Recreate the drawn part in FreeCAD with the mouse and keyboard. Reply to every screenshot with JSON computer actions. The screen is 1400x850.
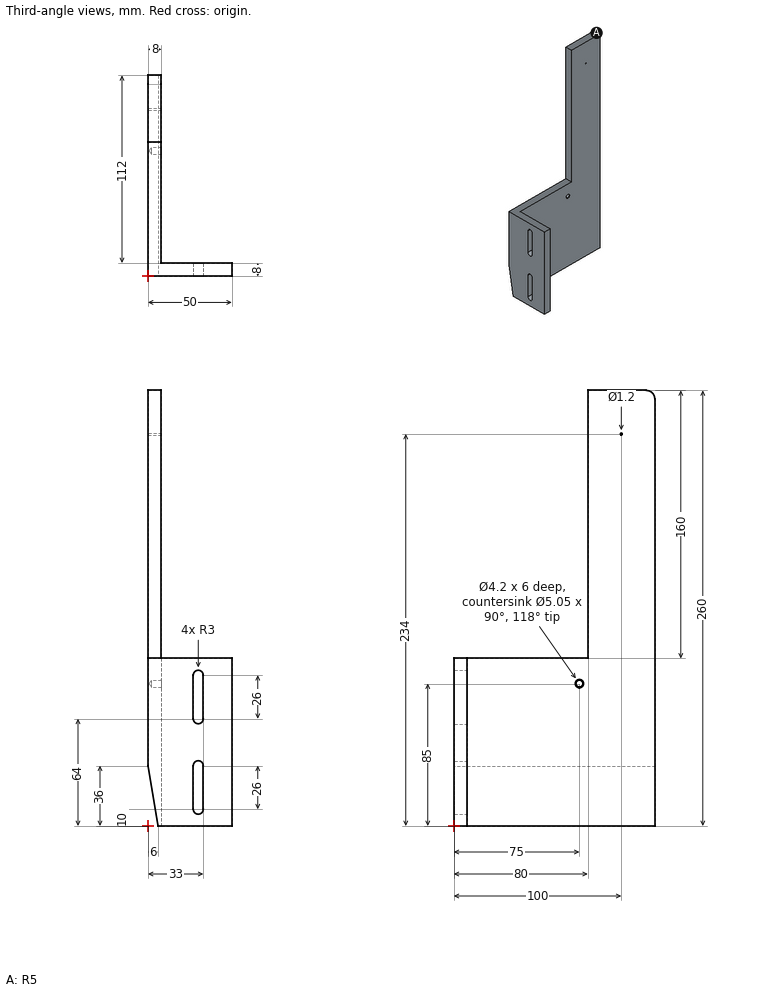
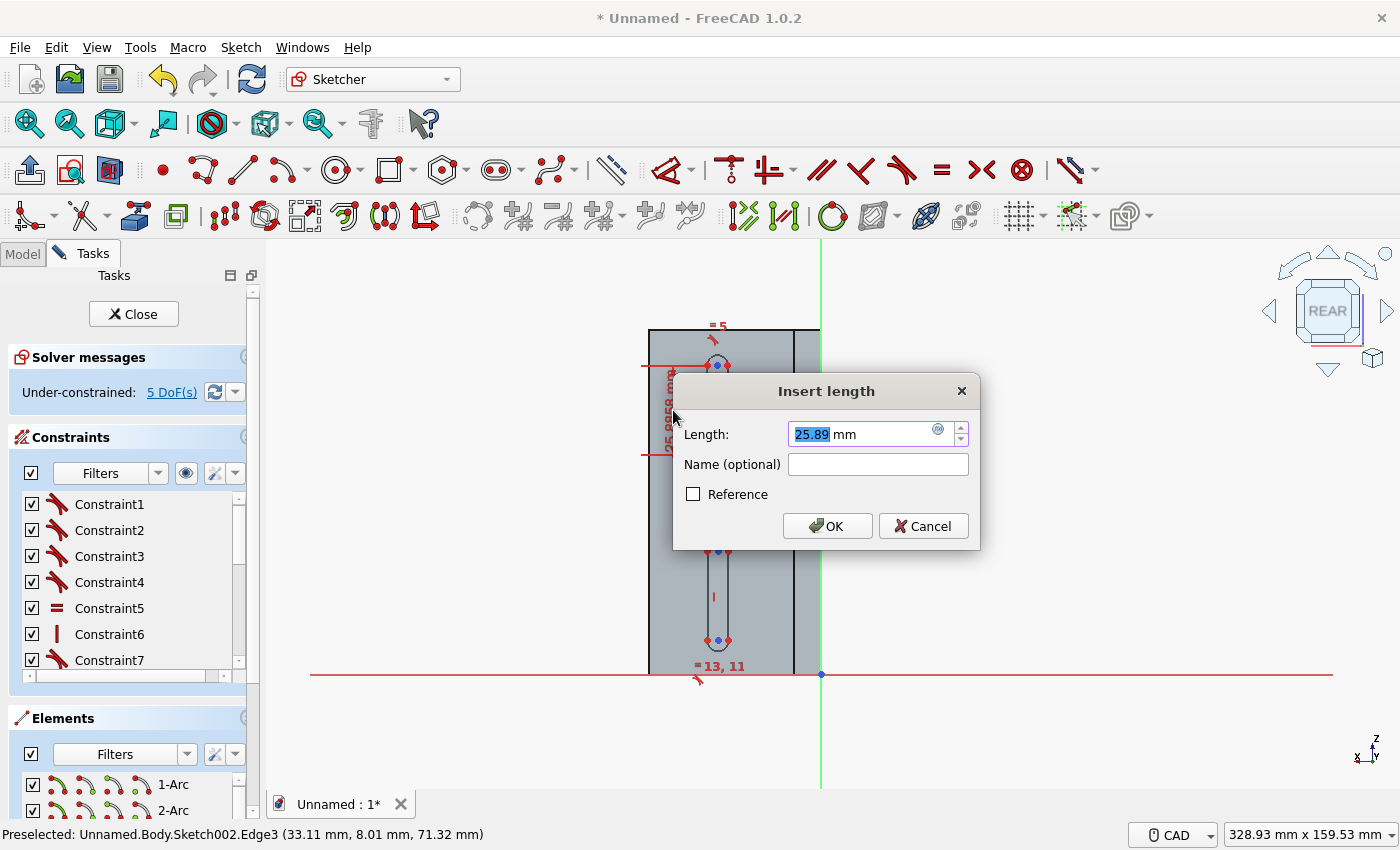
{"action": "type", "text": "26"}
{"action": "key", "text": "Return"}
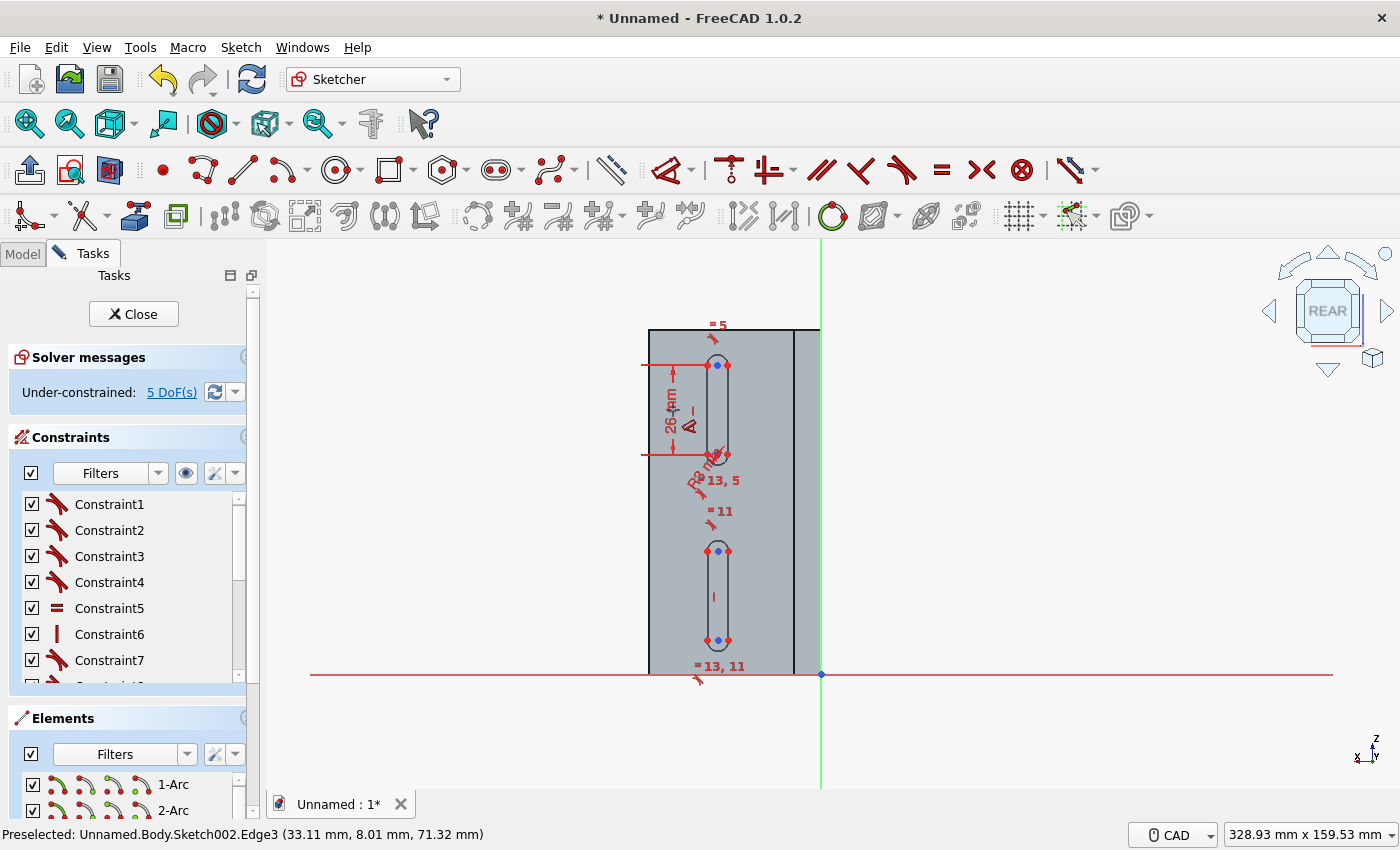
{"action": "left_click", "coordinate": [708, 614]}
{"action": "left_click", "coordinate": [674, 596]}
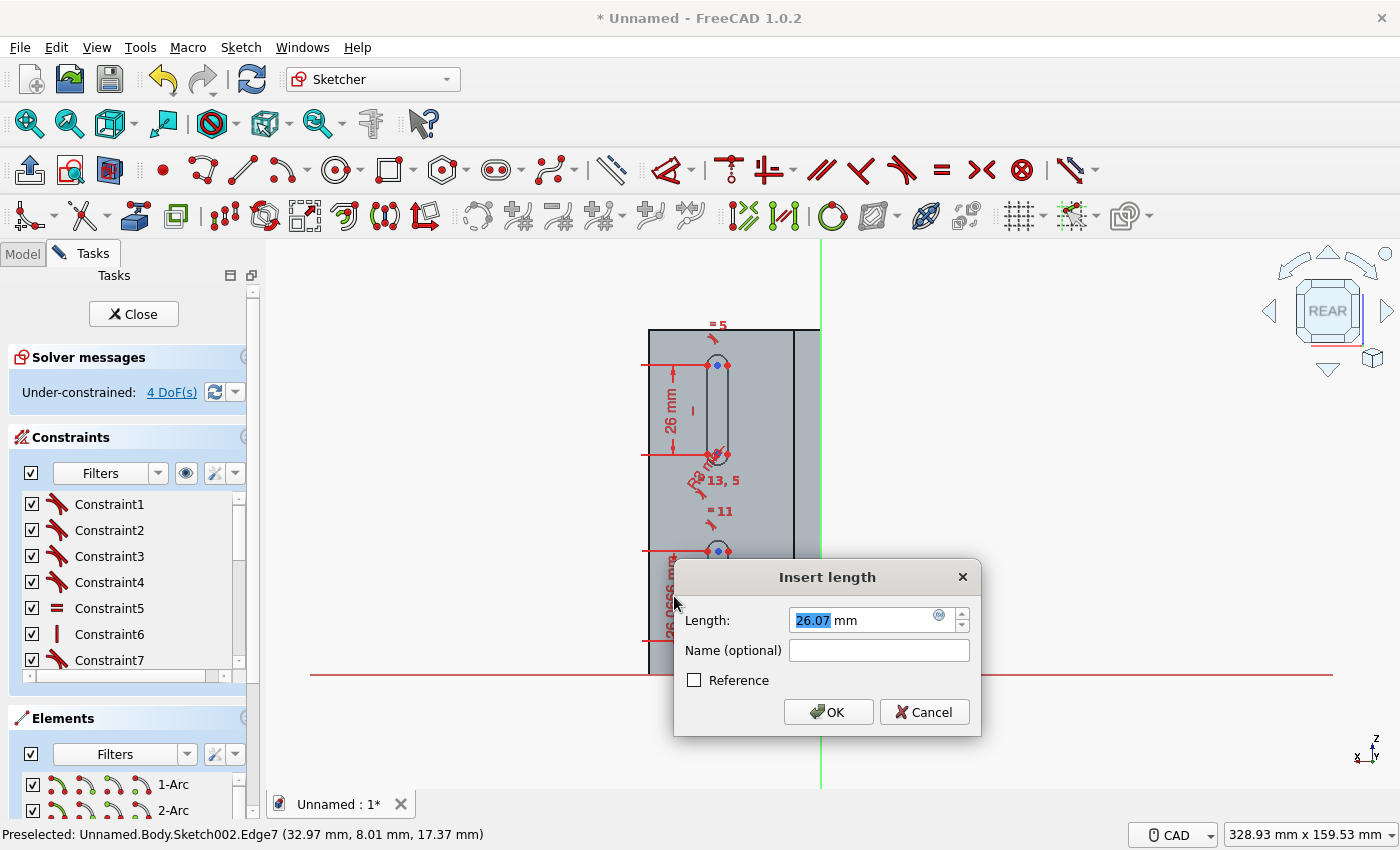
{"action": "type", "text": "26"}
{"action": "key", "text": "Return"}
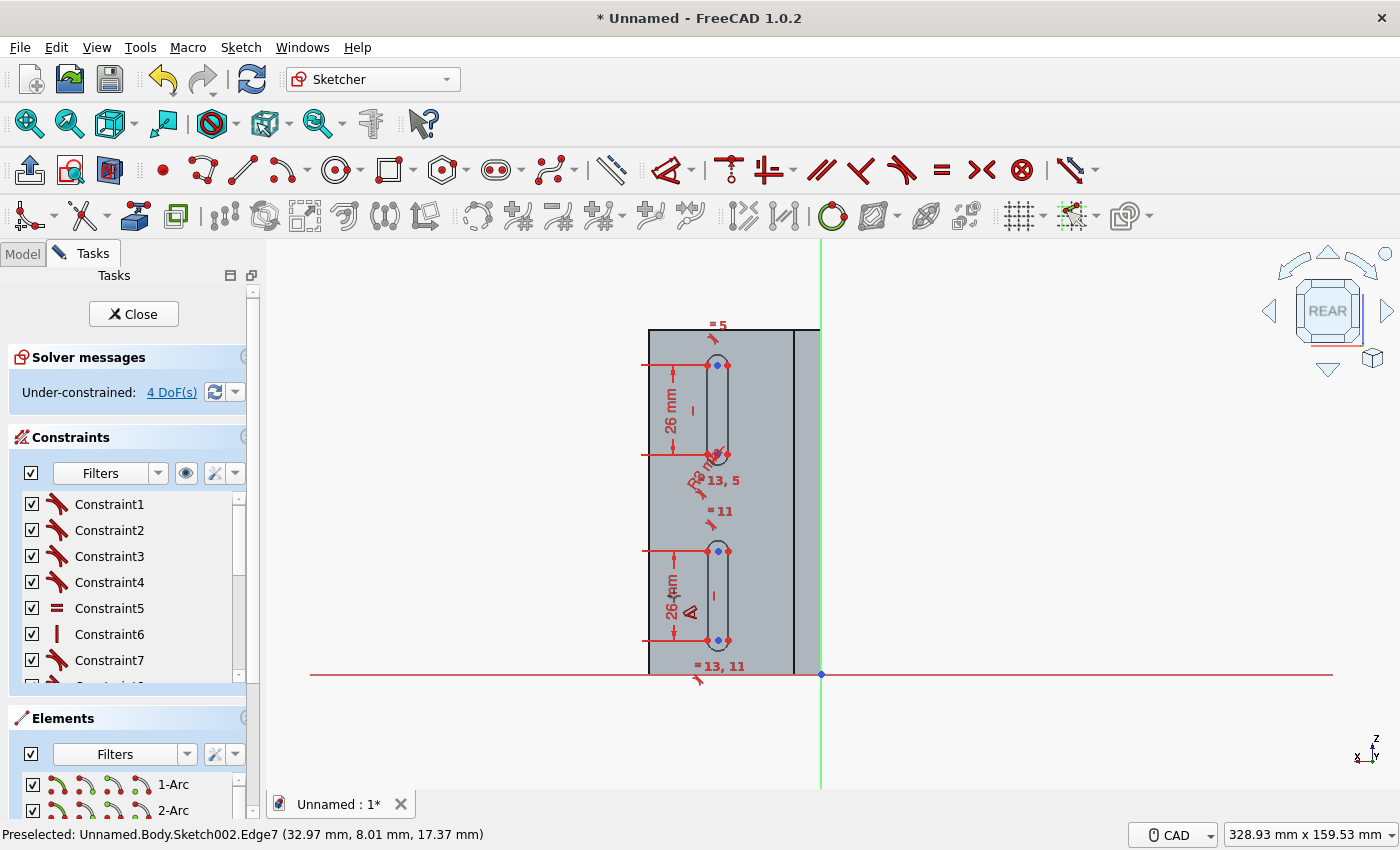
{"action": "left_click", "coordinate": [707, 455]}
{"action": "left_click", "coordinate": [764, 709]}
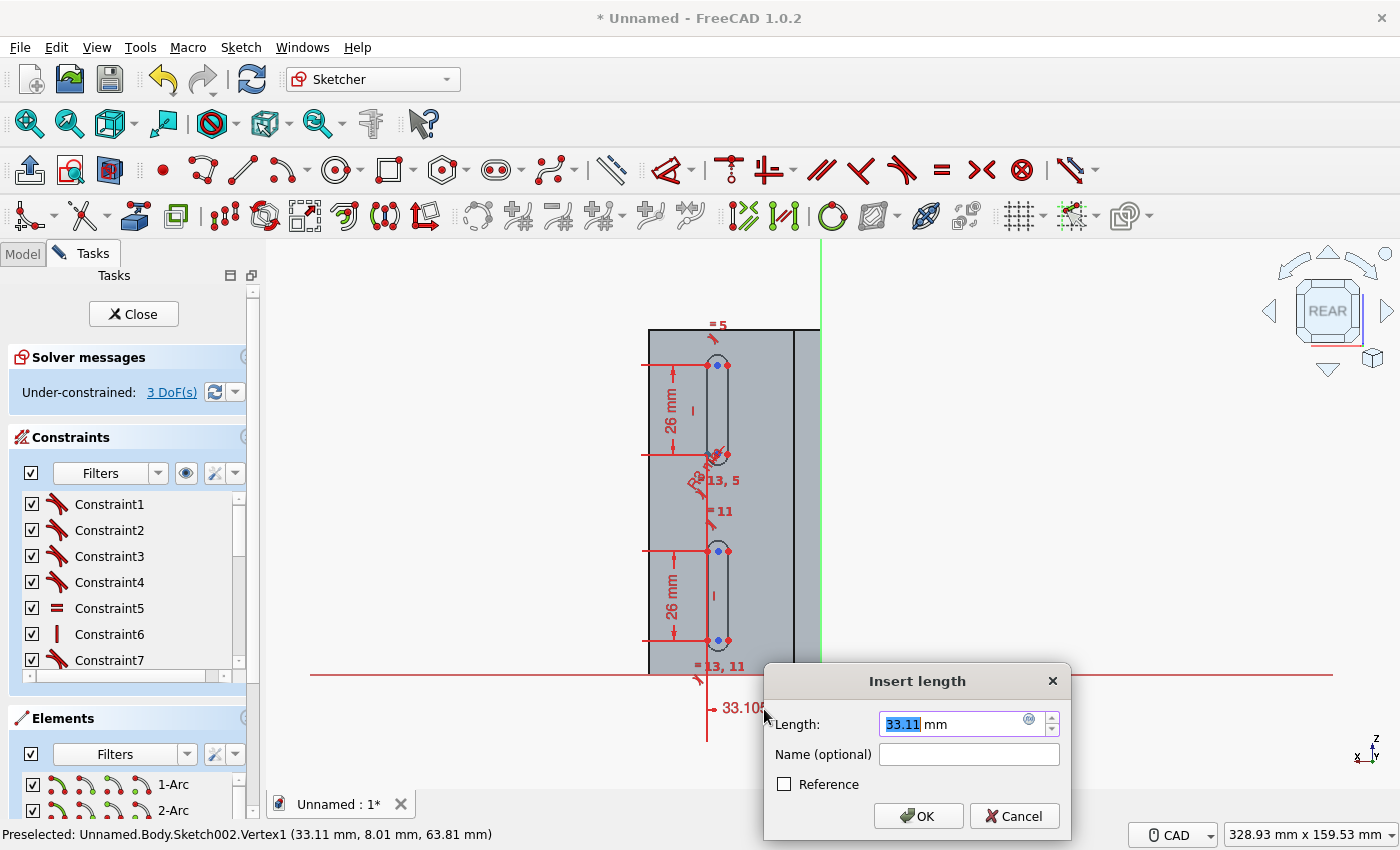
{"action": "type", "text": "33"}
{"action": "key", "text": "Return"}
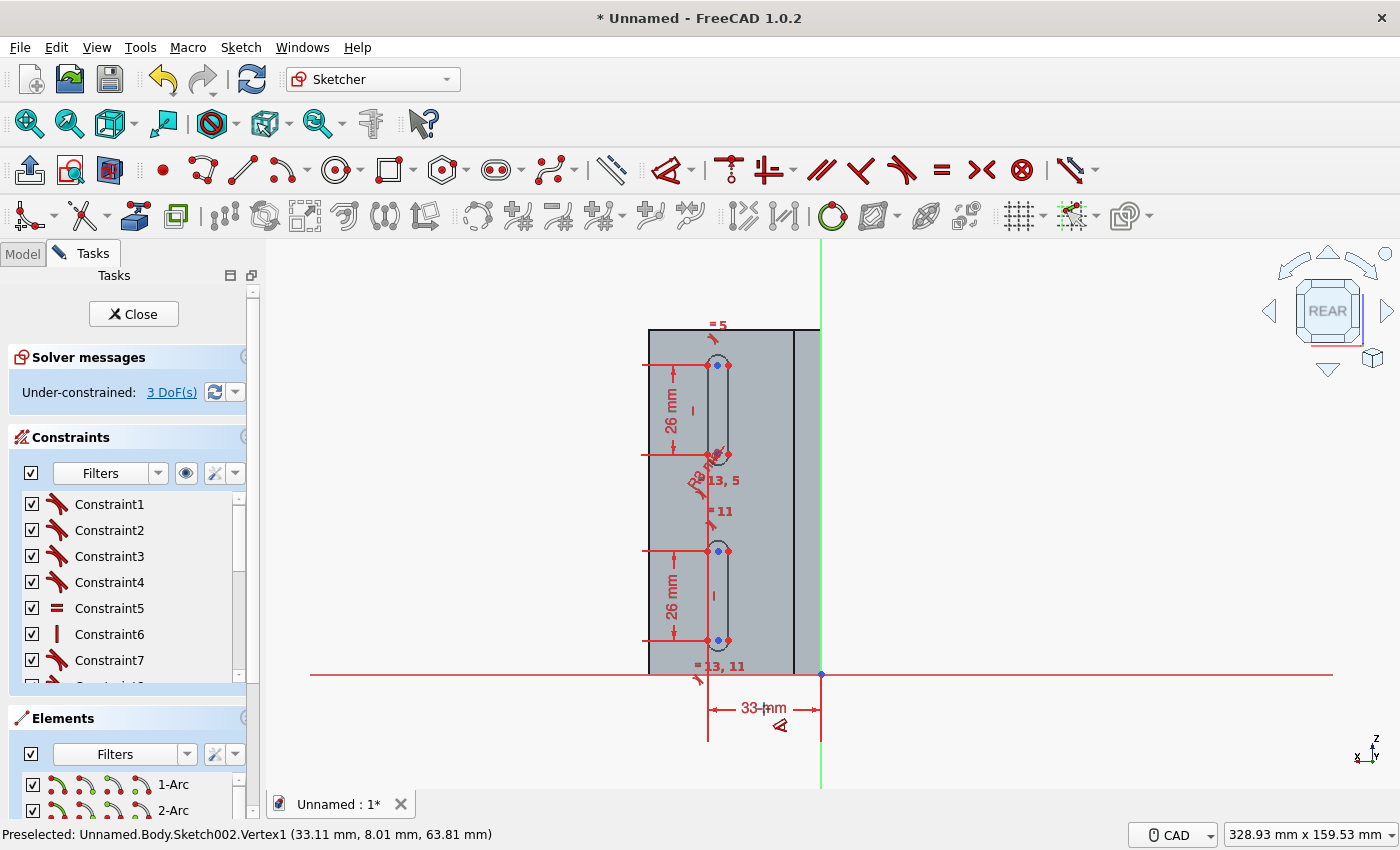
{"action": "left_click", "coordinate": [708, 455]}
{"action": "left_click", "coordinate": [674, 565]}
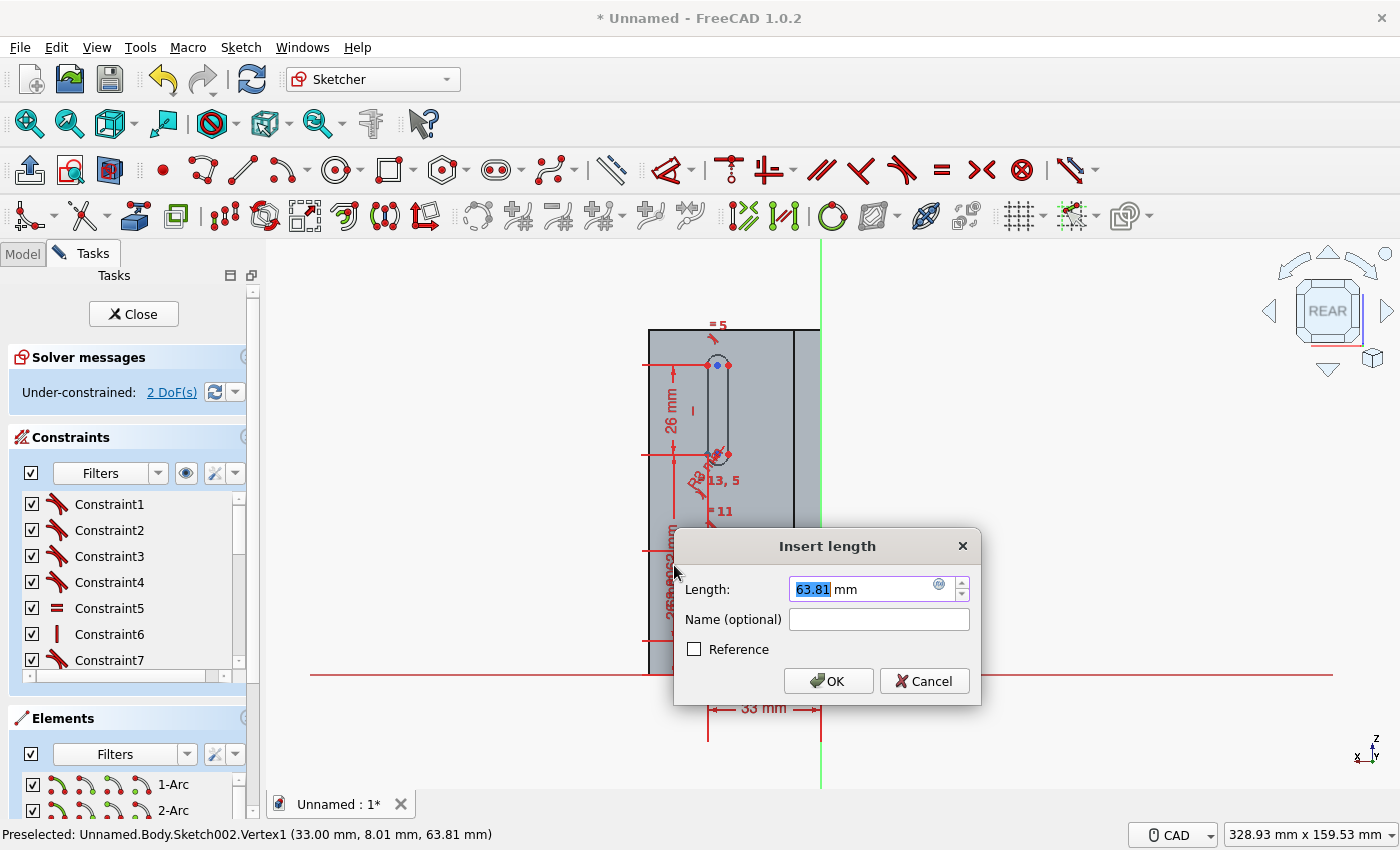
{"action": "type", "text": "64"}
{"action": "key", "text": "Return"}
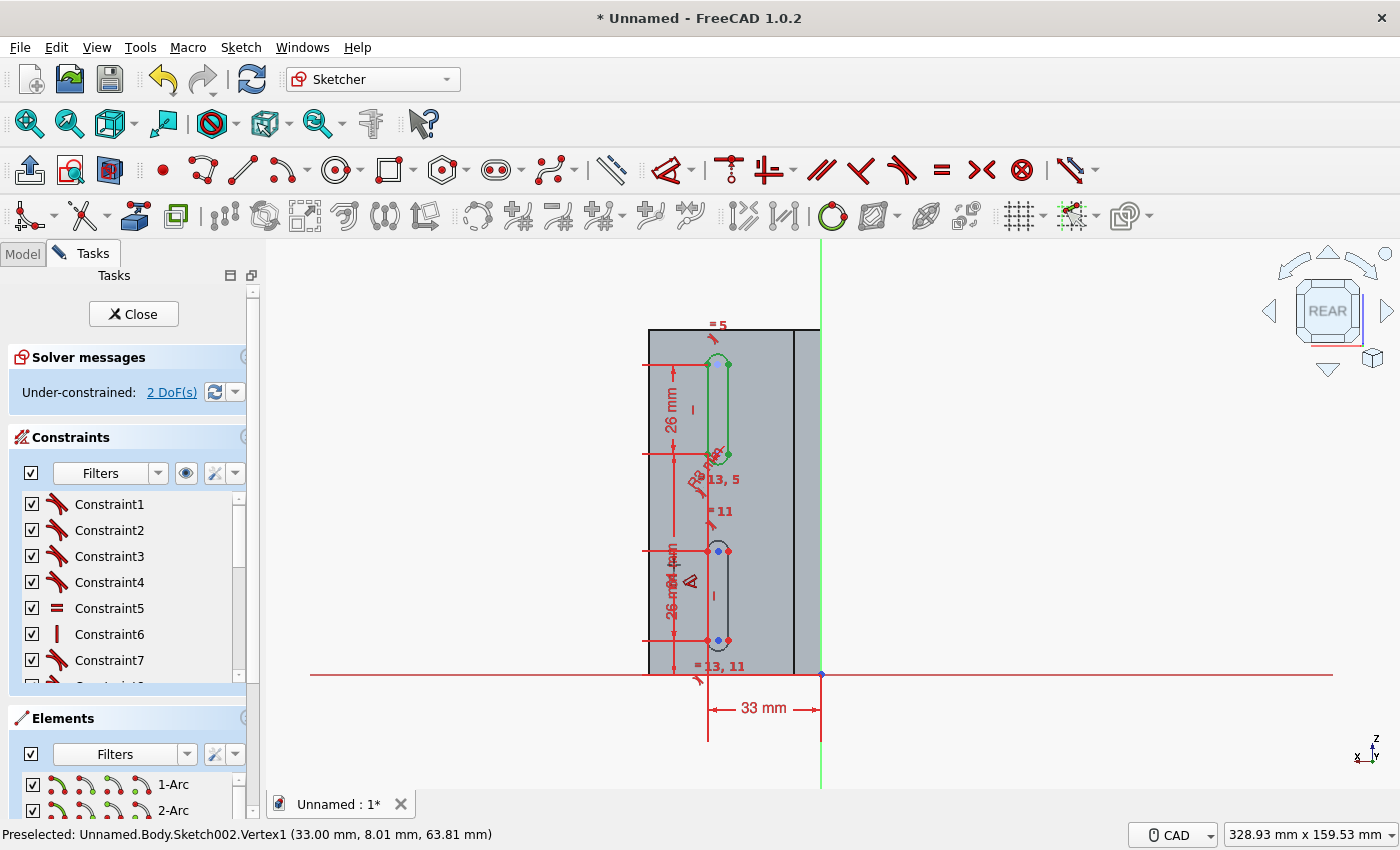
{"action": "left_click", "coordinate": [708, 641]}
{"action": "left_click", "coordinate": [765, 607]}